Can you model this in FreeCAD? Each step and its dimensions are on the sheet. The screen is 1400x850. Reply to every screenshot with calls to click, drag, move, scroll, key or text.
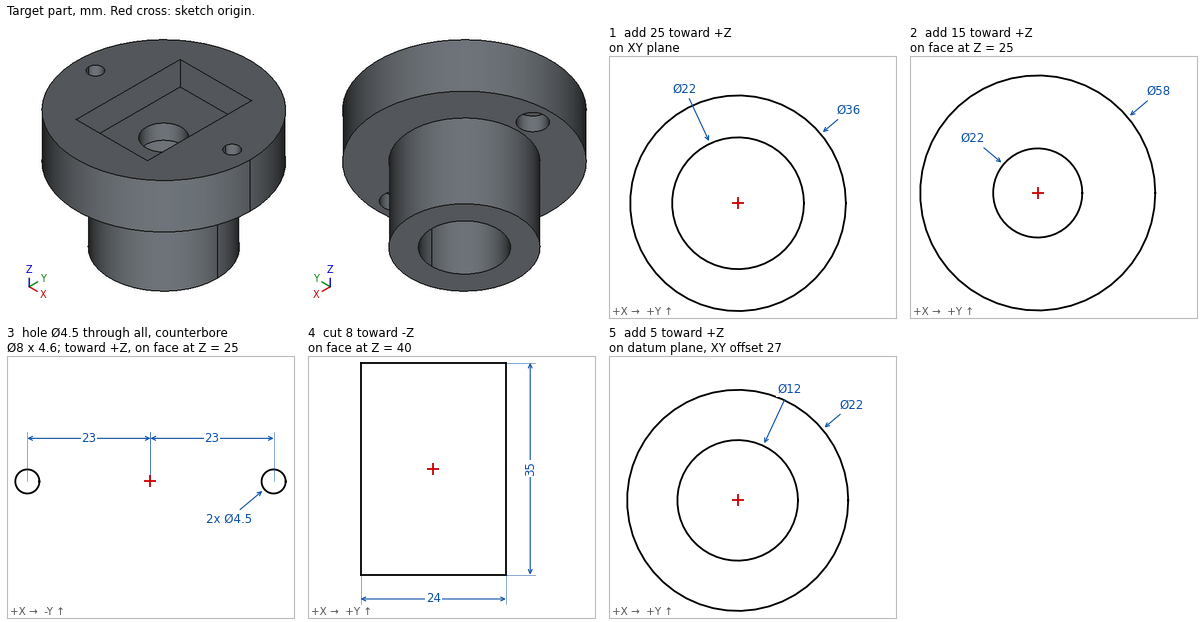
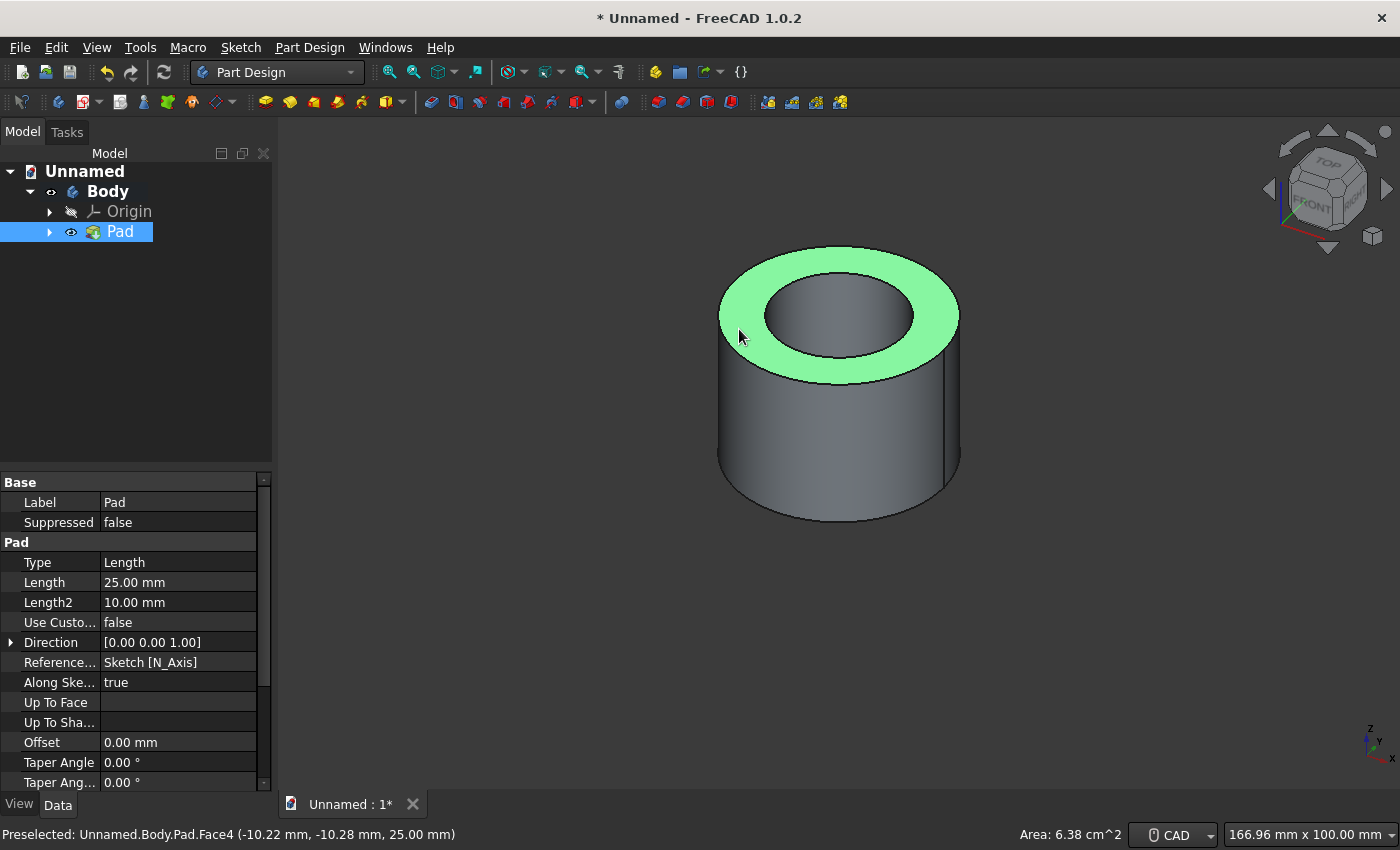
click(84, 102)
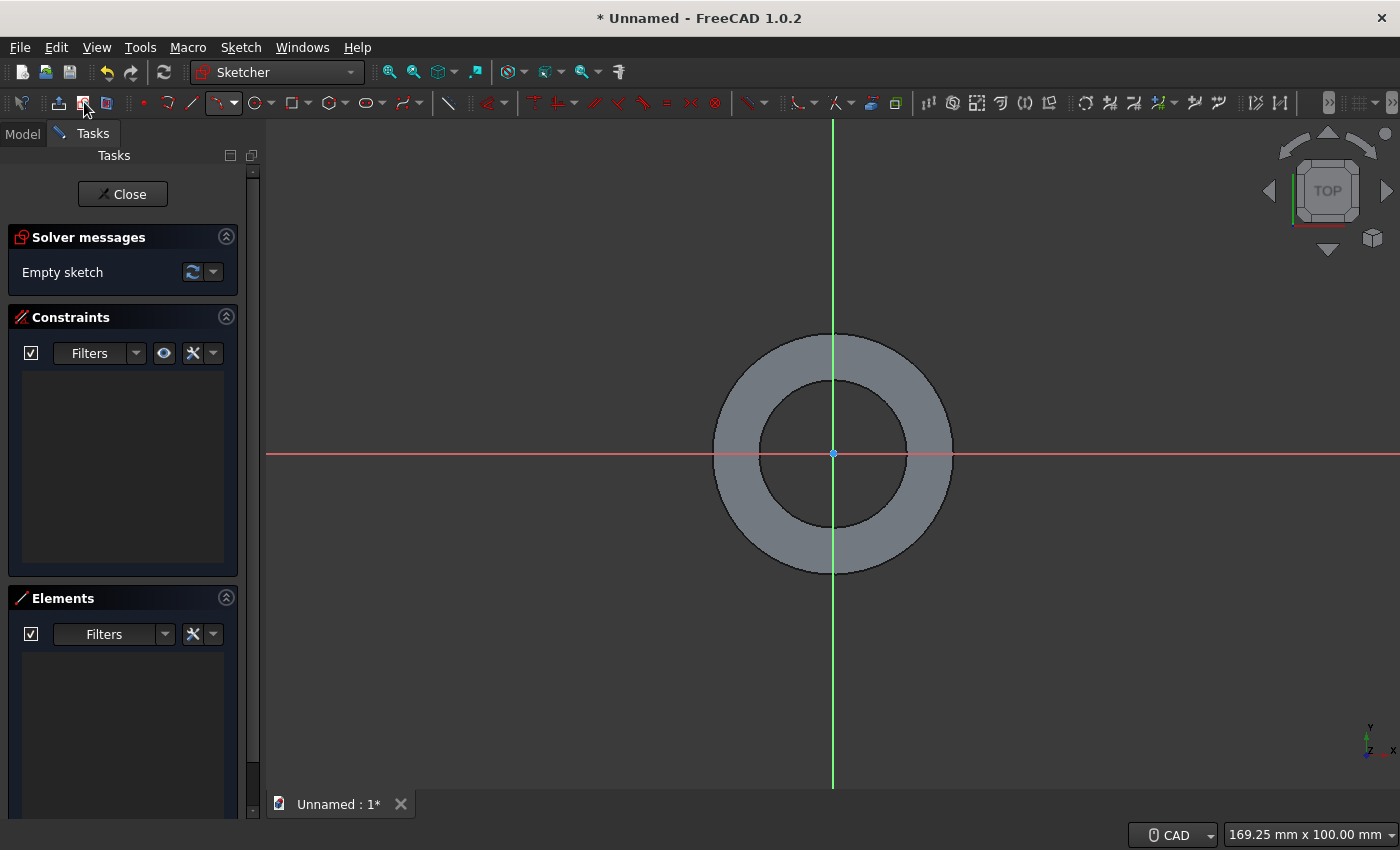
key(g)
key(c)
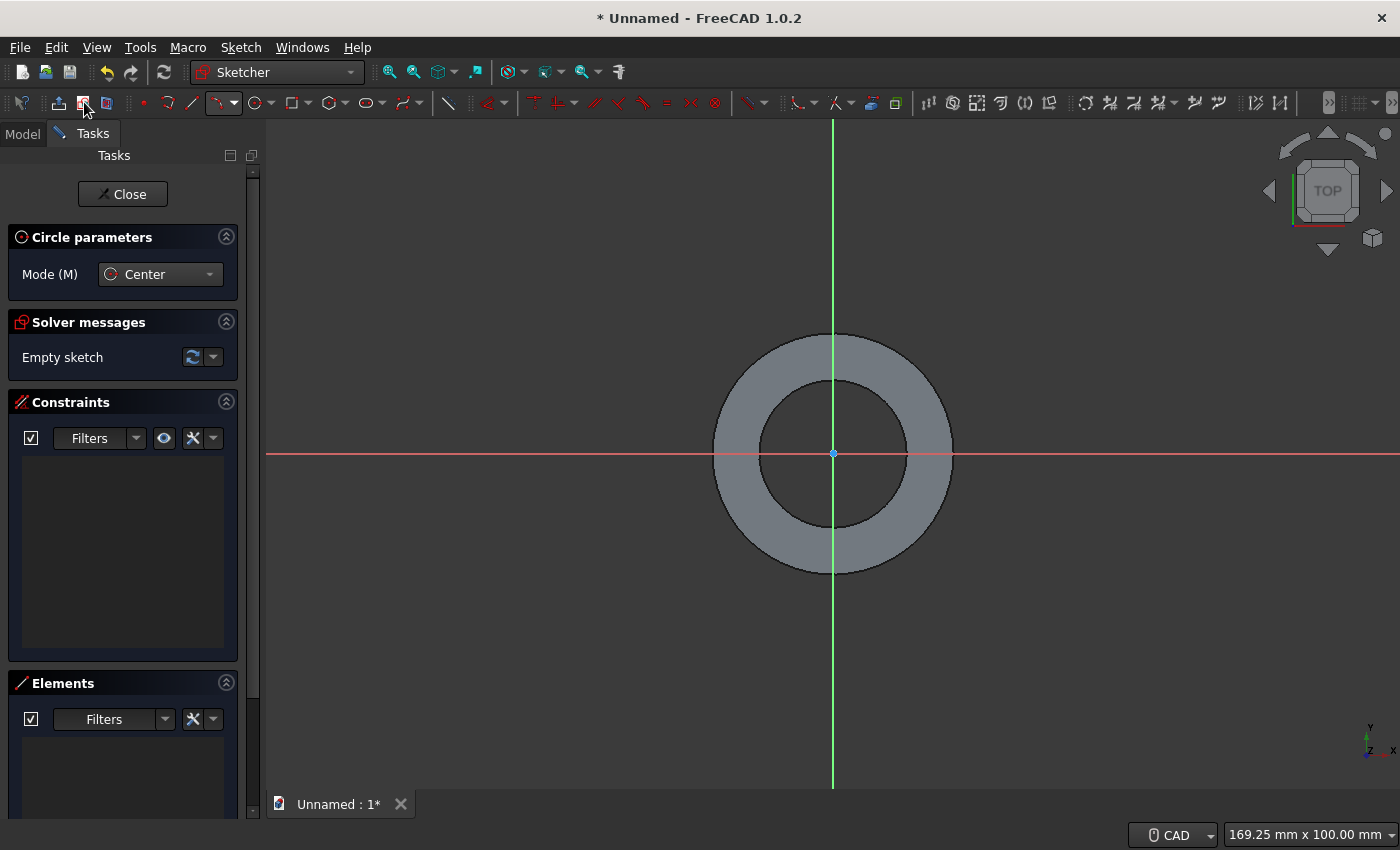
click(833, 454)
click(970, 317)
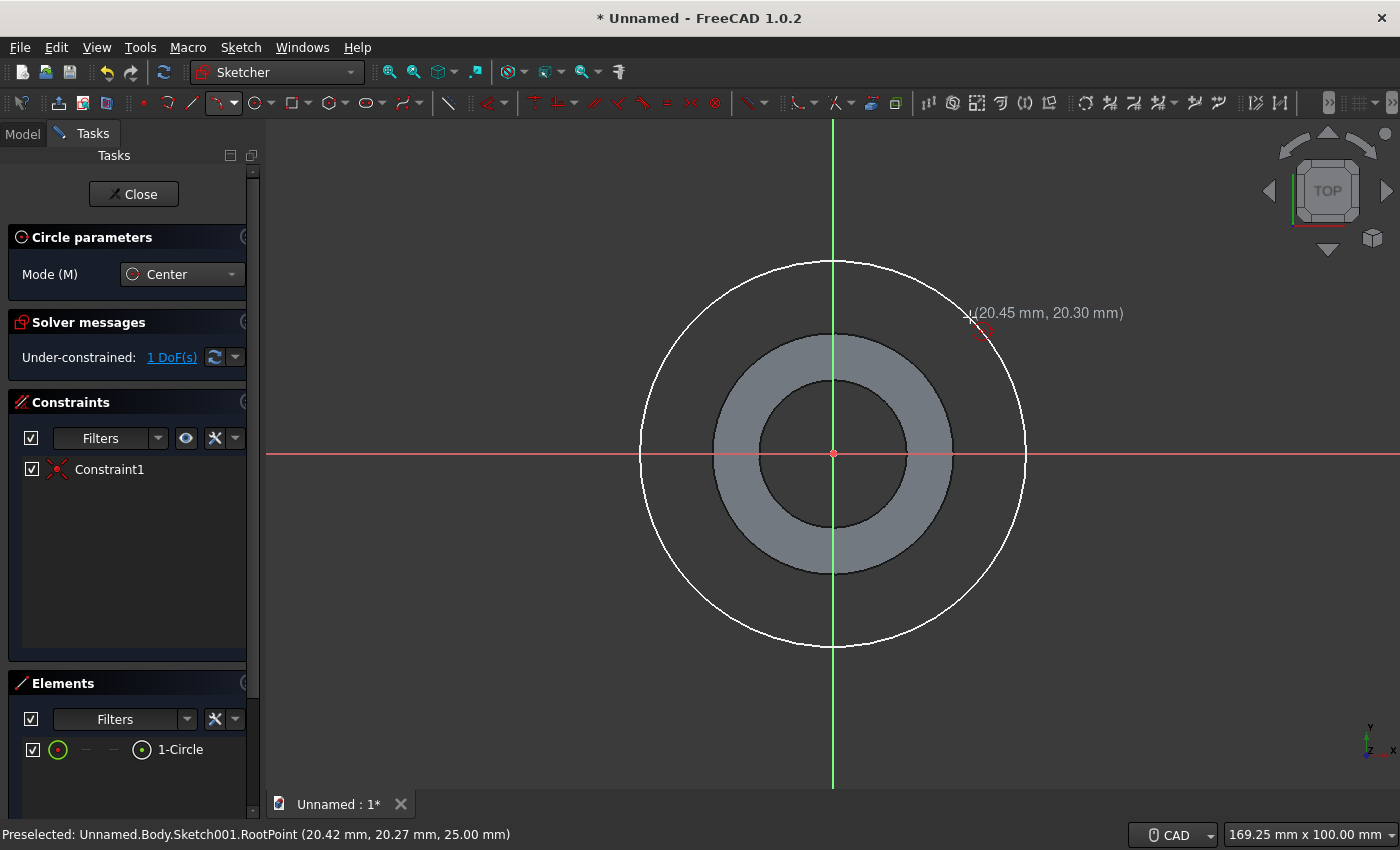
click(833, 454)
click(885, 402)
key(Escape)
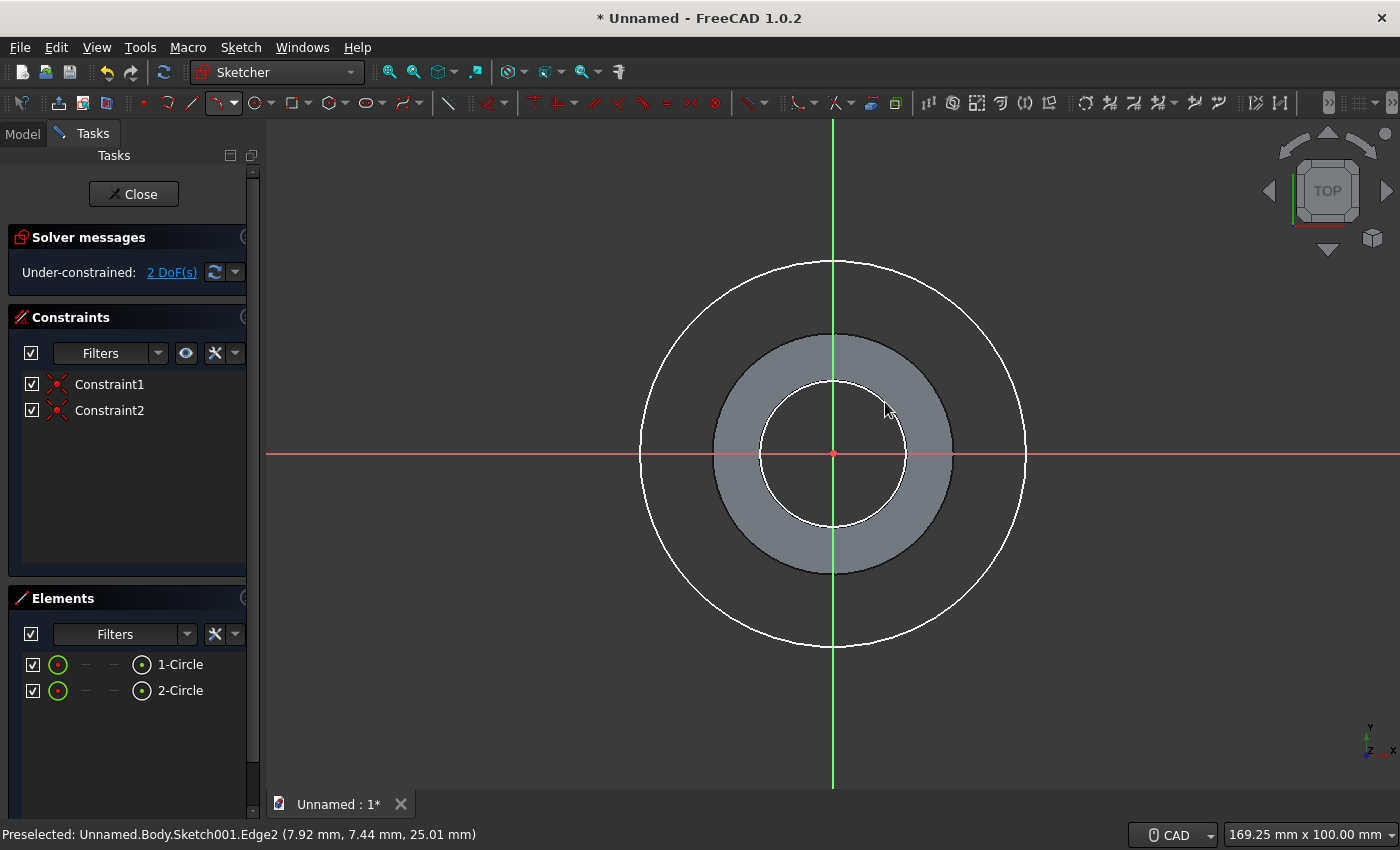
key(d)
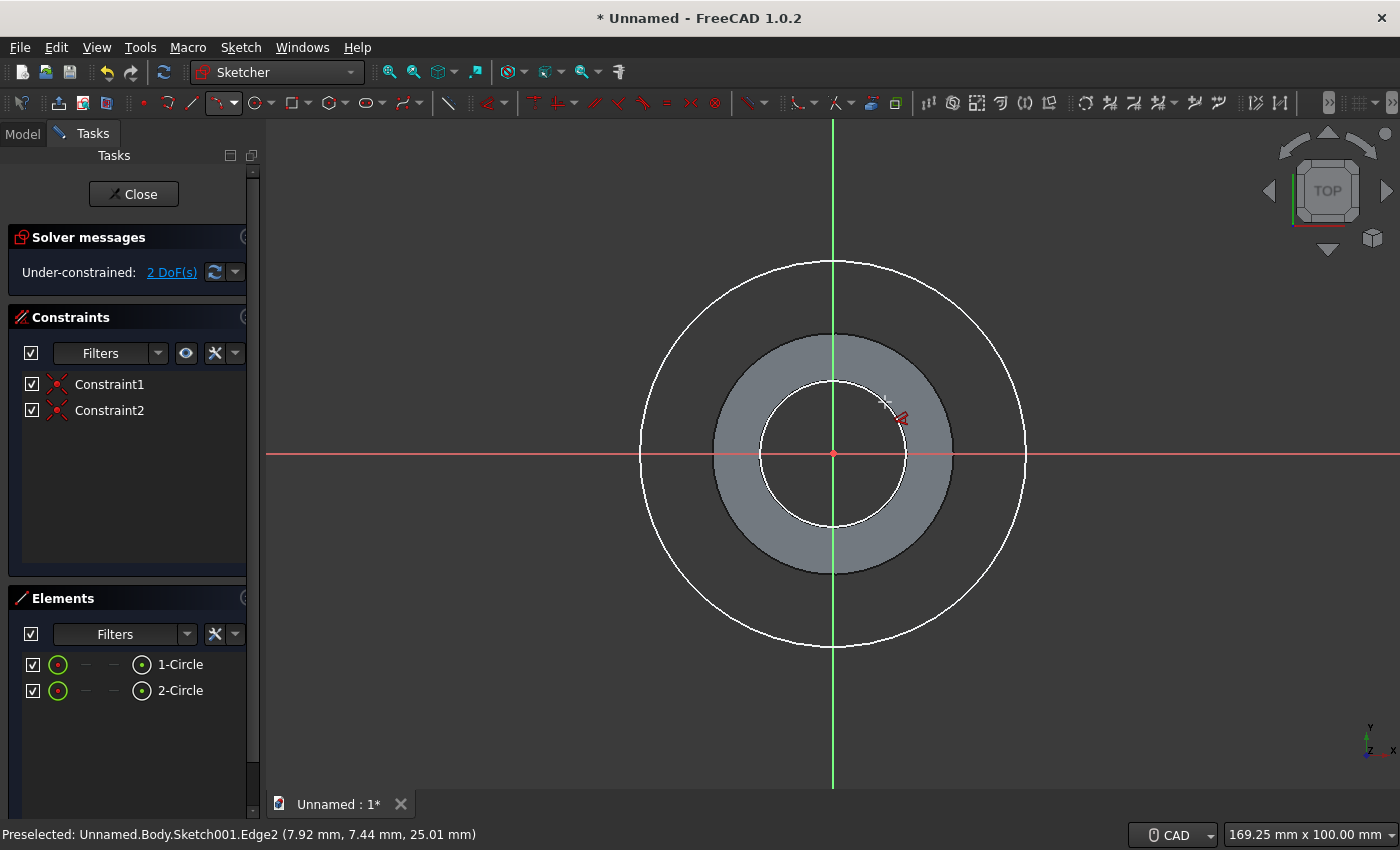
click(969, 317)
click(992, 294)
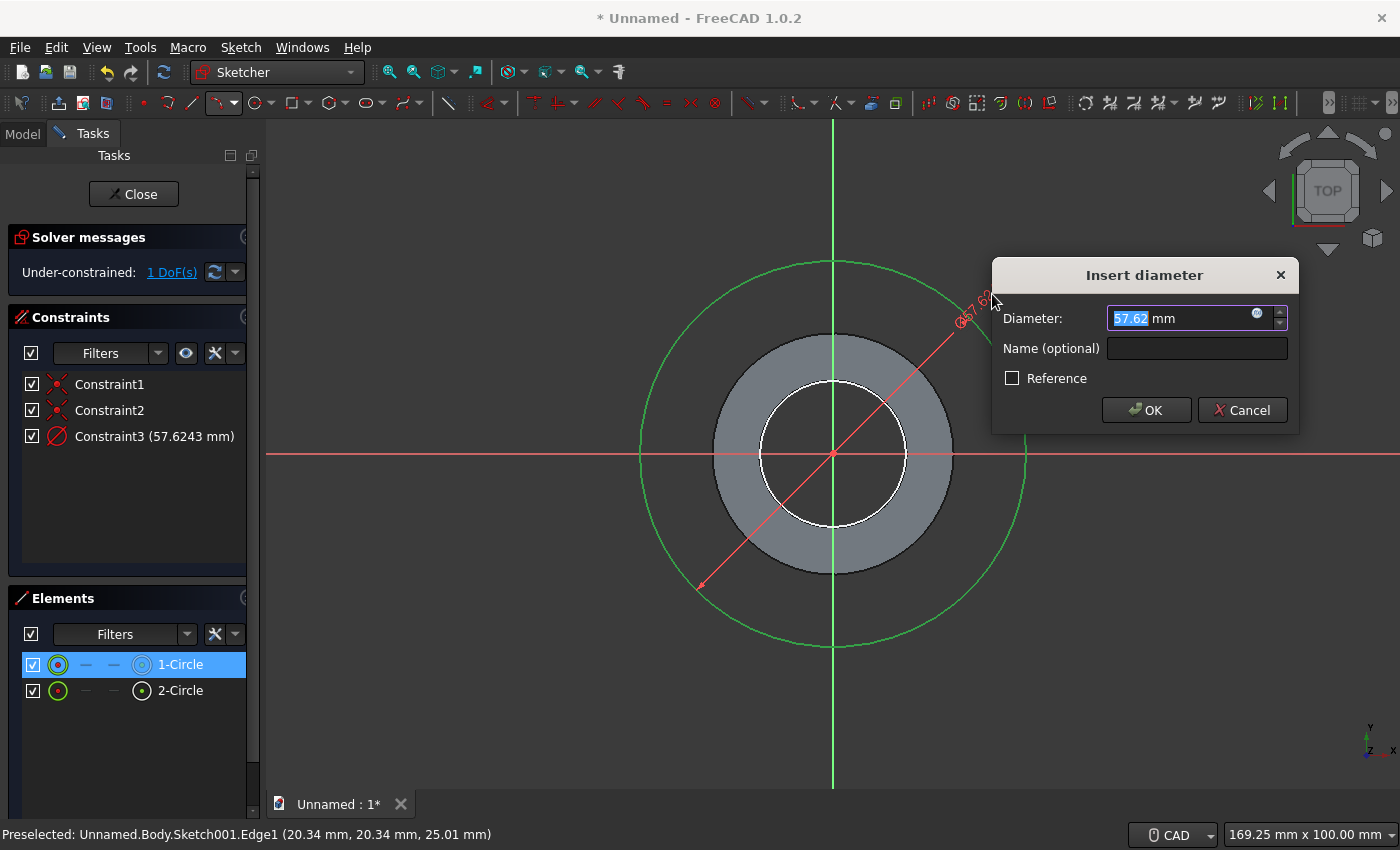
text(58)
key(Return)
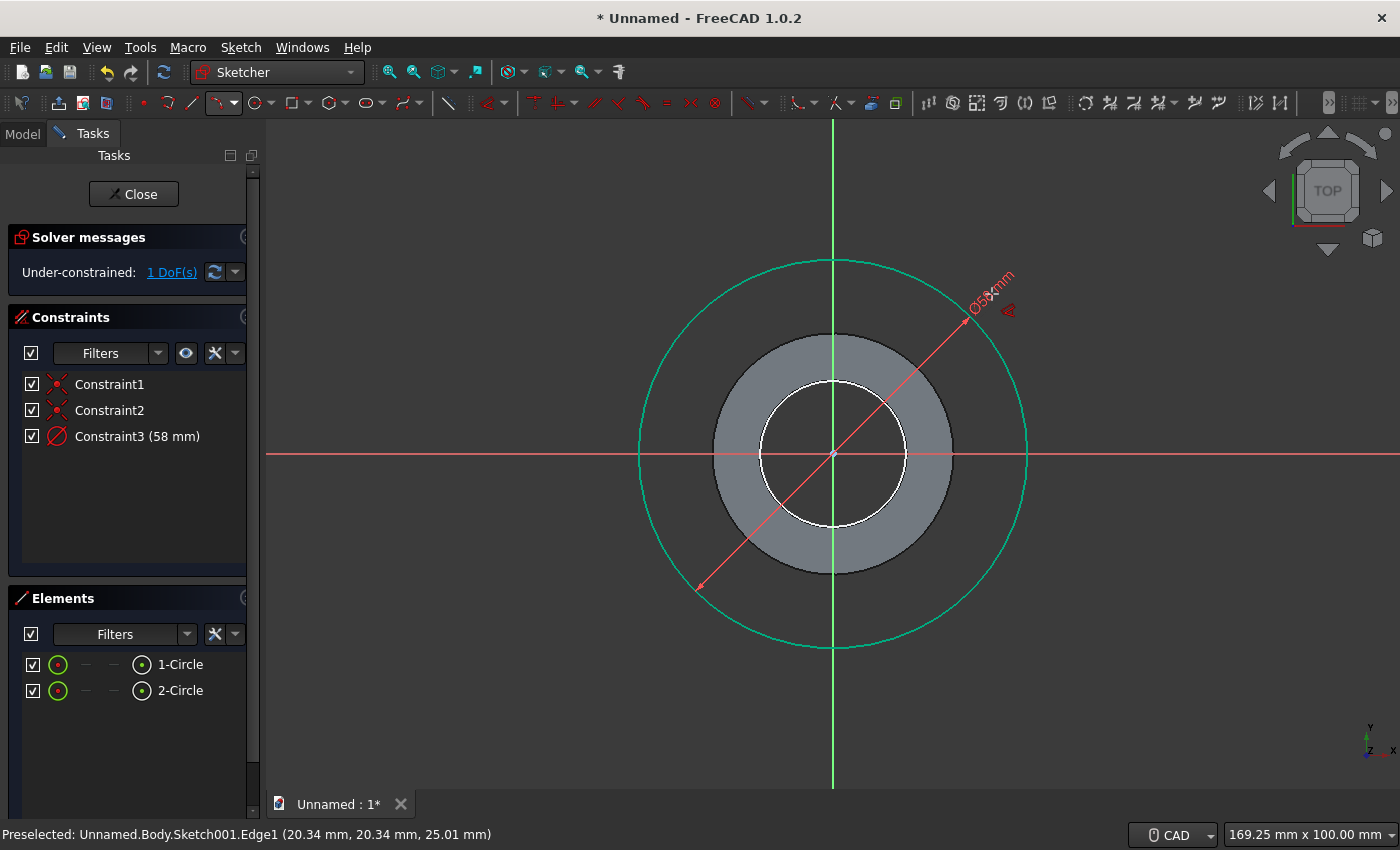
click(884, 402)
click(906, 379)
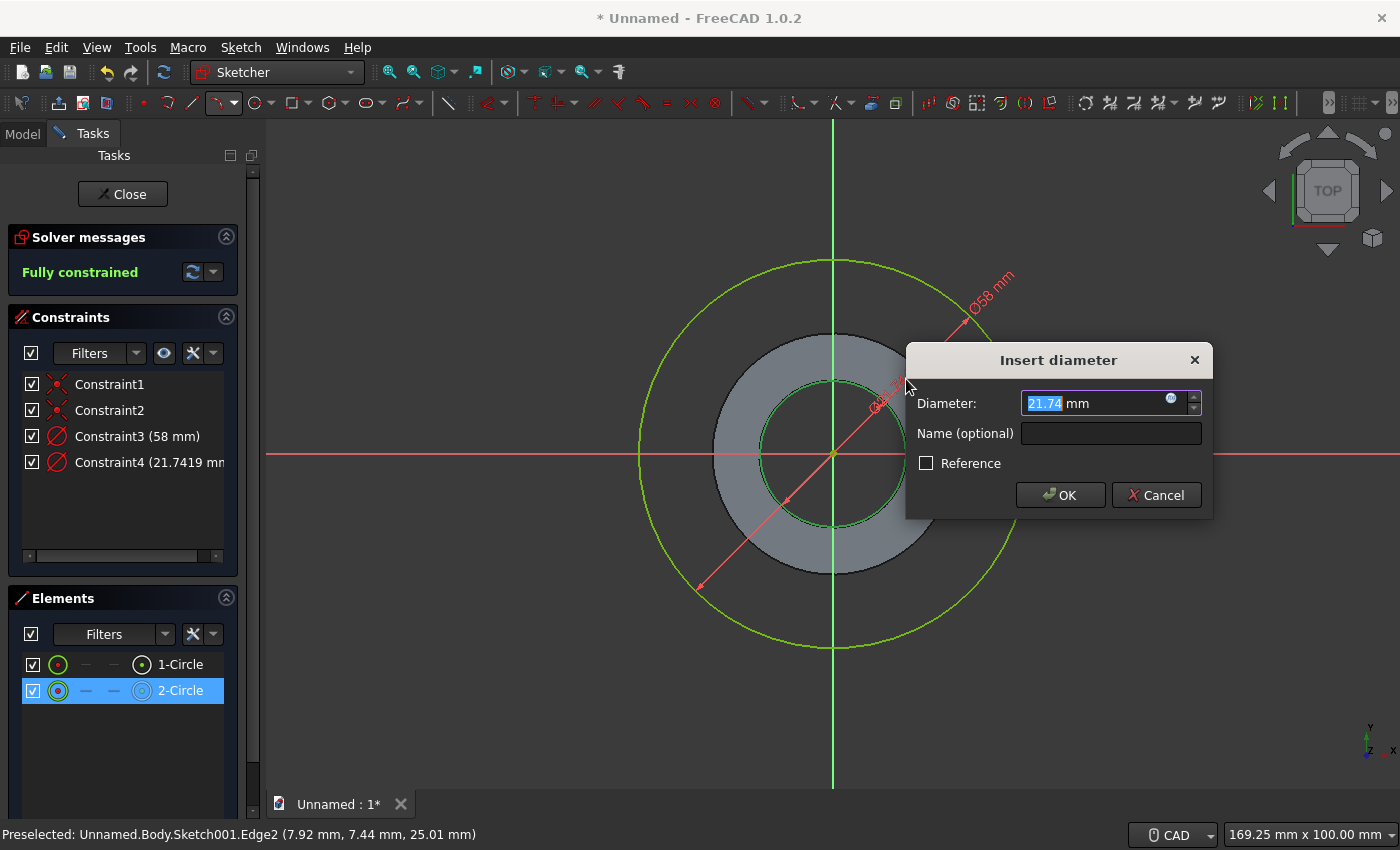
text(22)
key(Return)
key(Escape)